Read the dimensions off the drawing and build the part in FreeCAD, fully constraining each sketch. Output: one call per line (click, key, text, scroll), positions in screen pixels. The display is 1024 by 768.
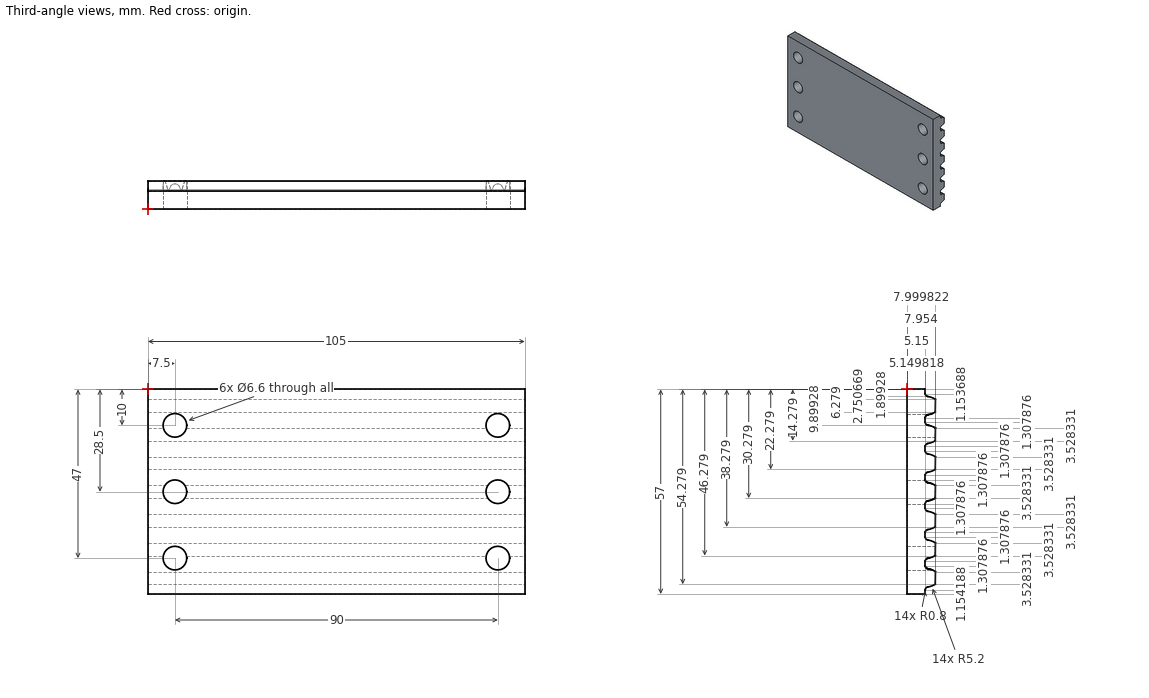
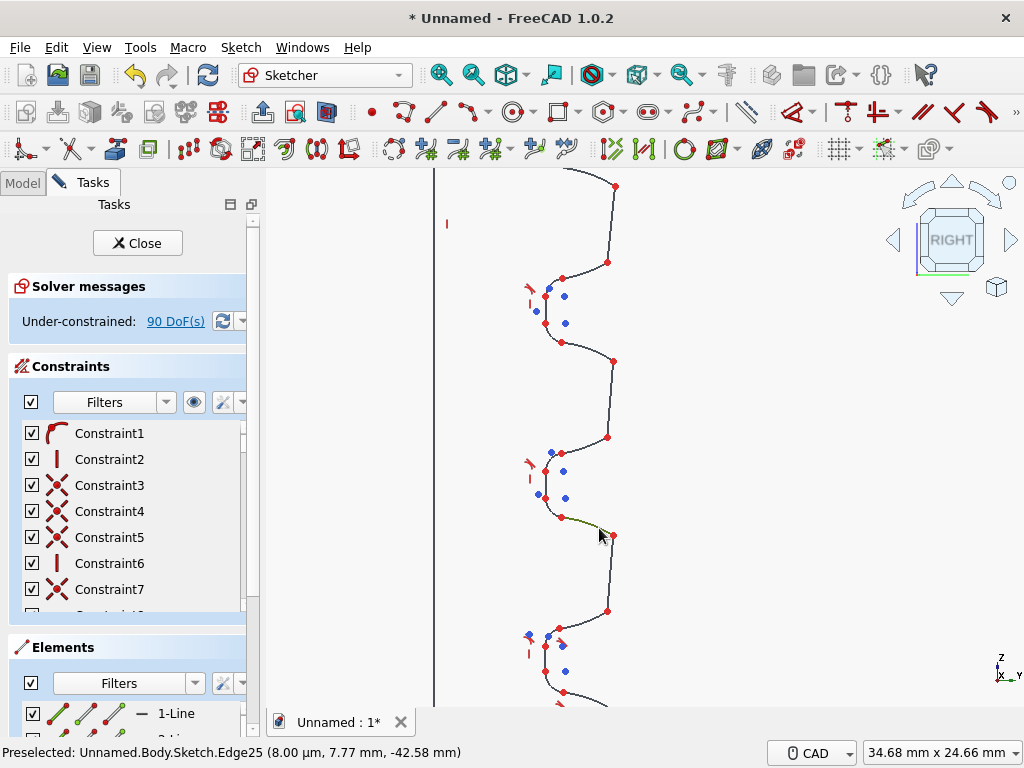
click(550, 510)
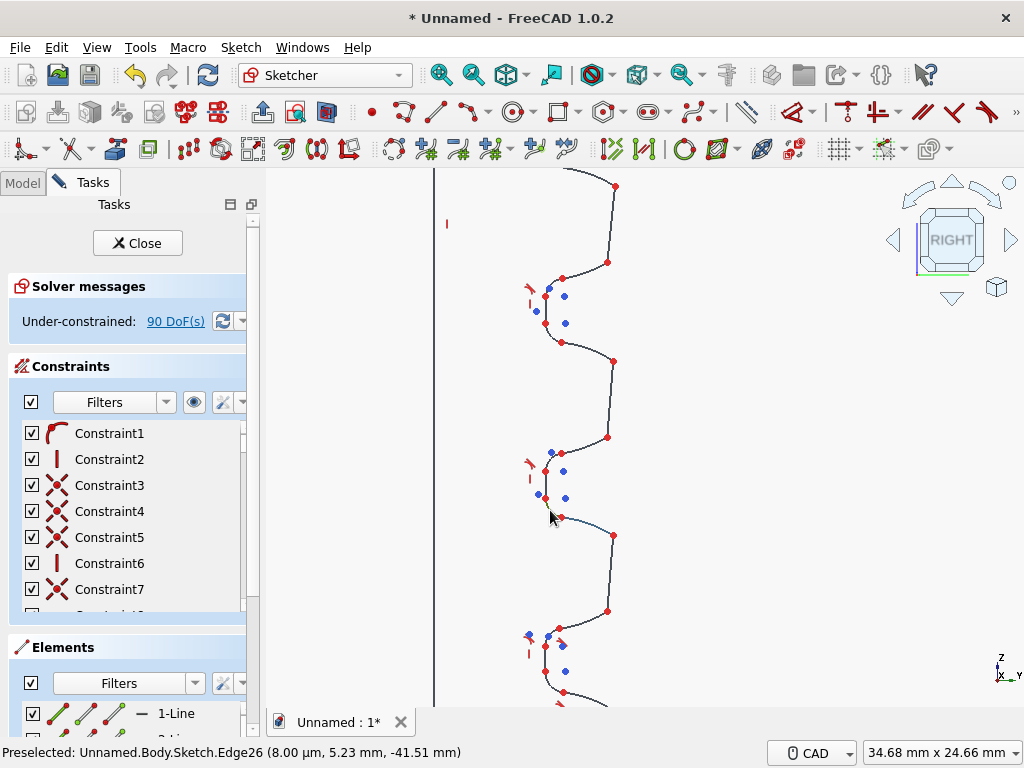
click(988, 112)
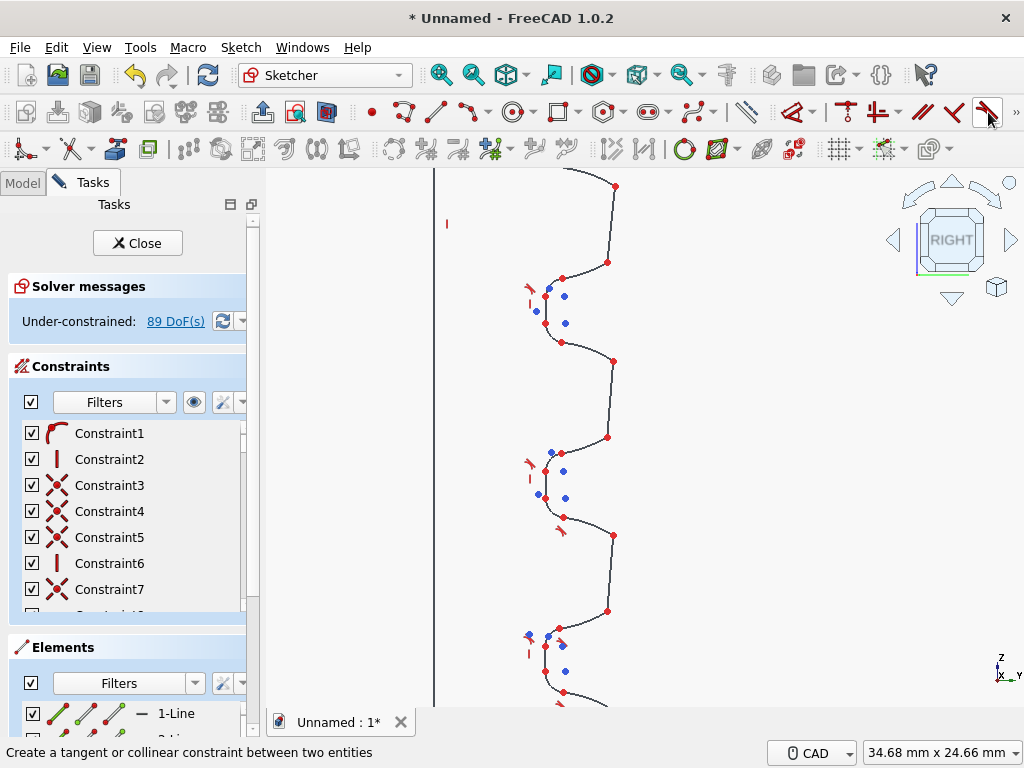
click(550, 459)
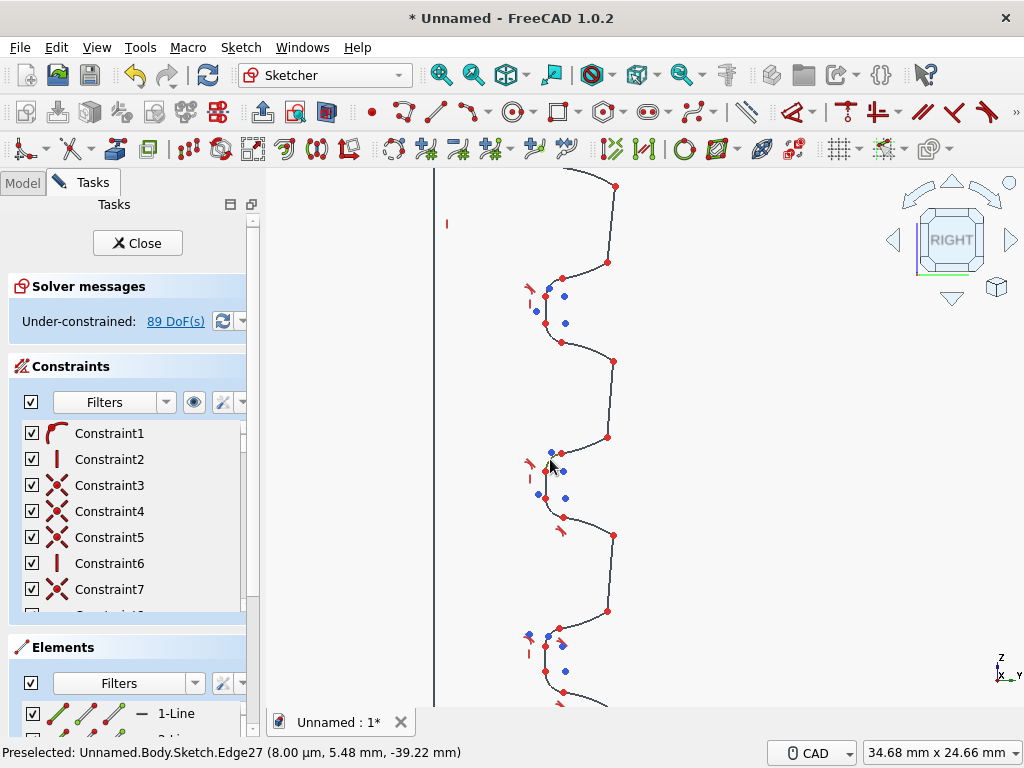
click(576, 450)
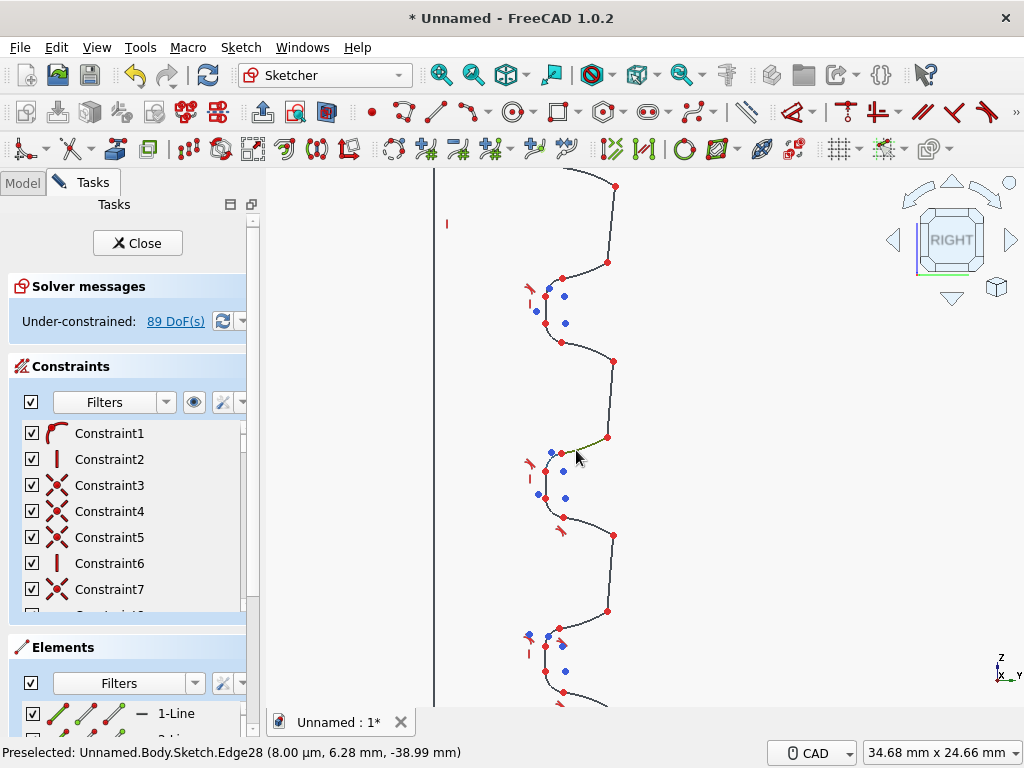
click(988, 112)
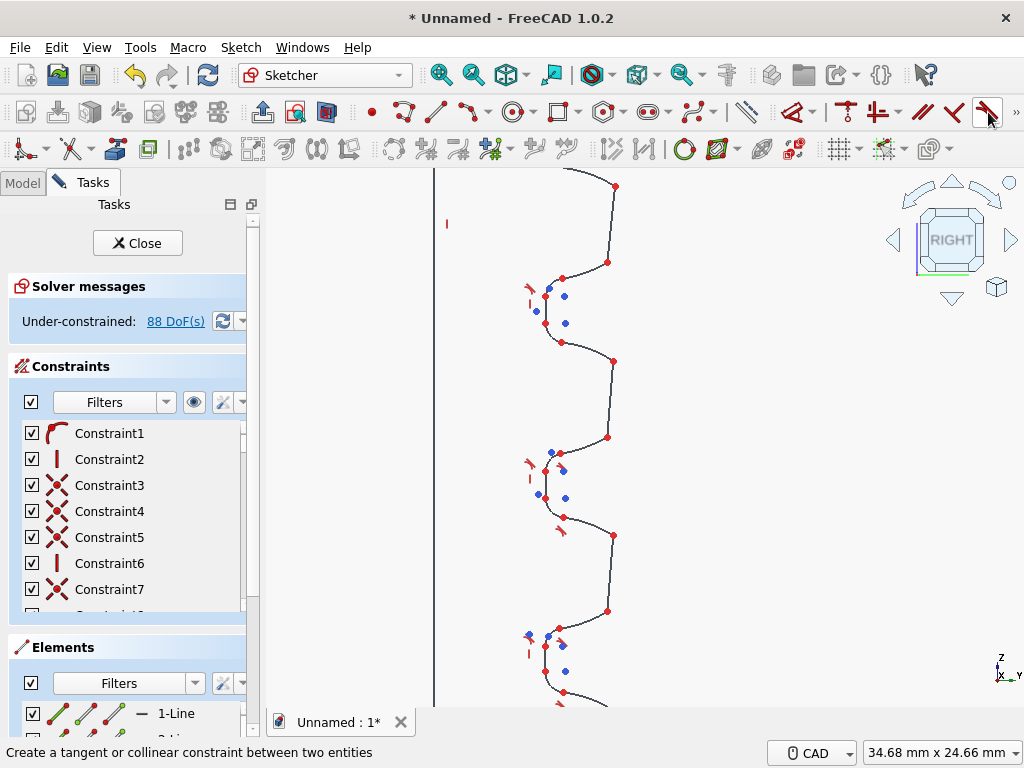
click(599, 353)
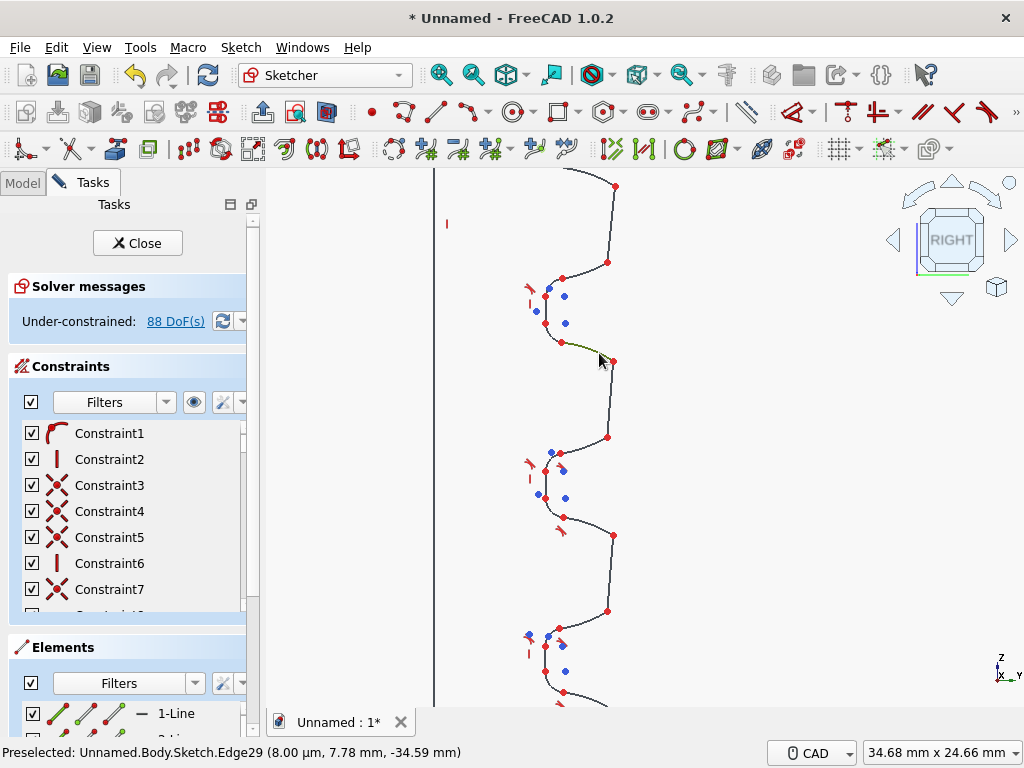
click(550, 336)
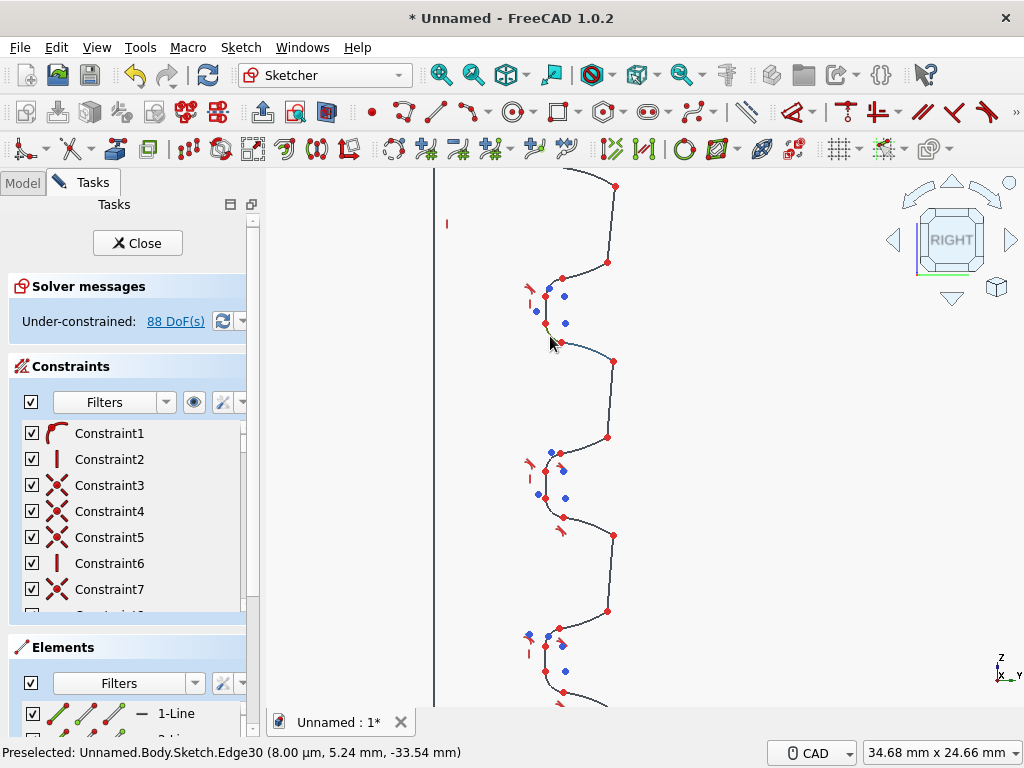
click(988, 112)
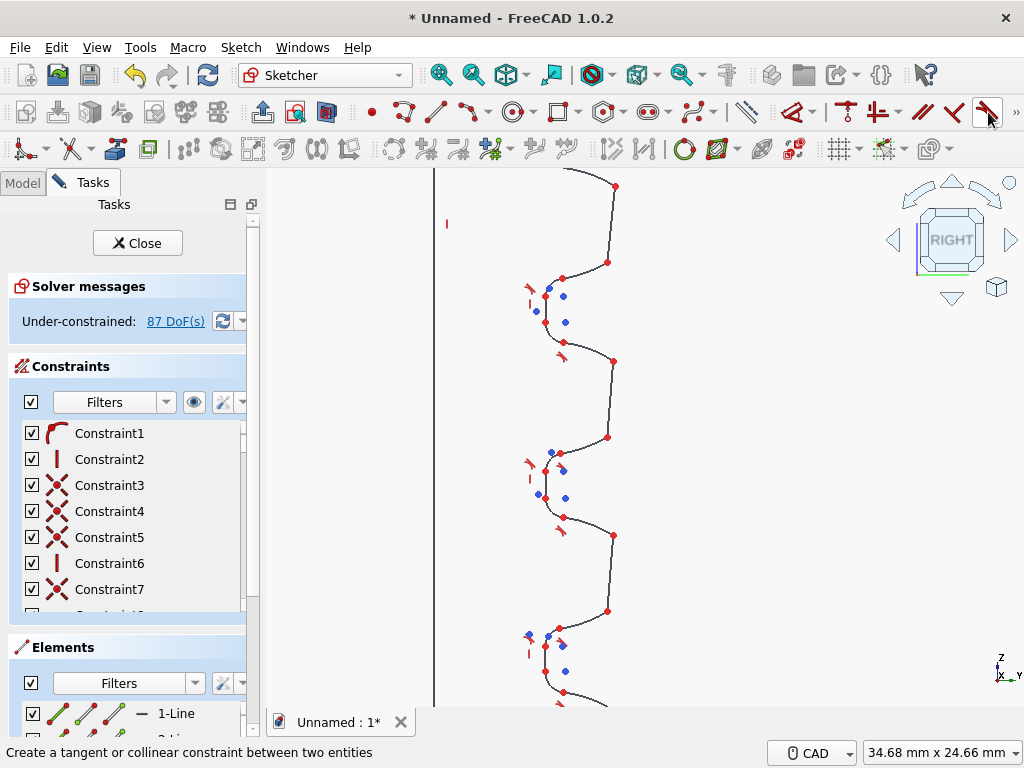
click(555, 281)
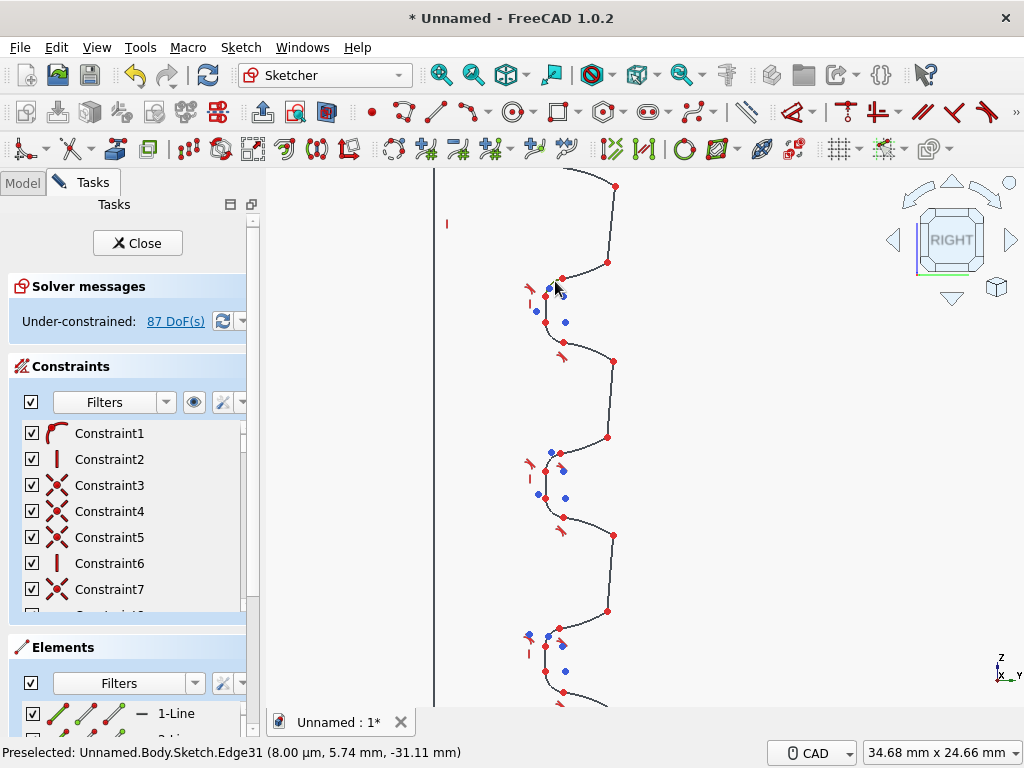
click(576, 276)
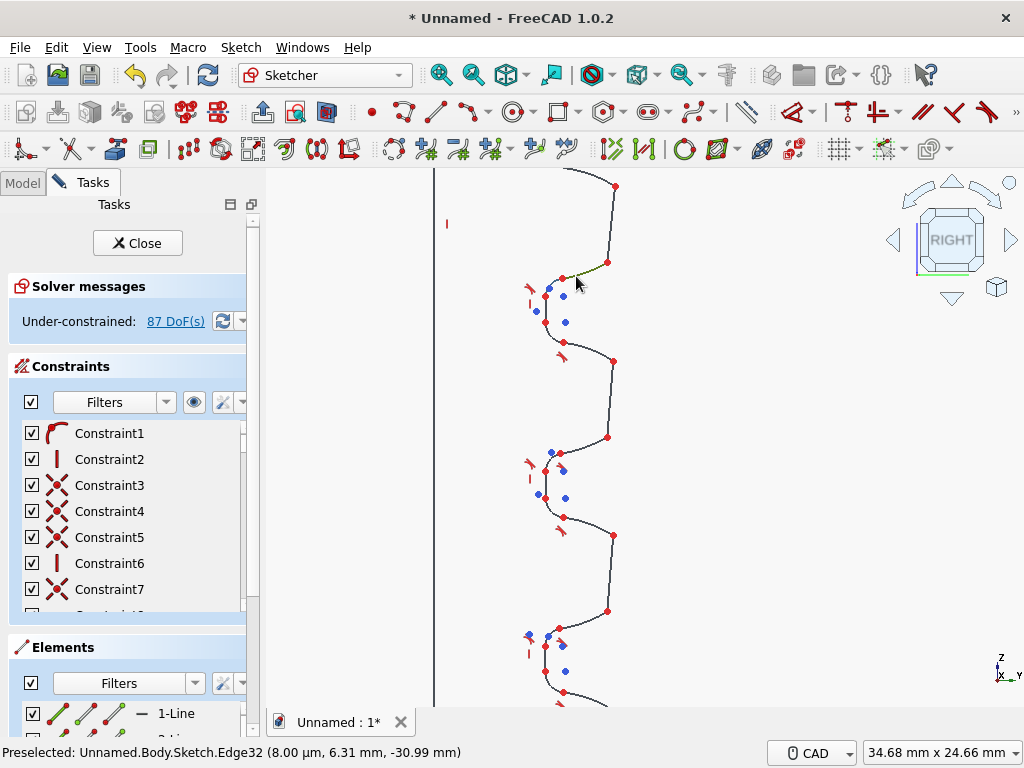
click(988, 112)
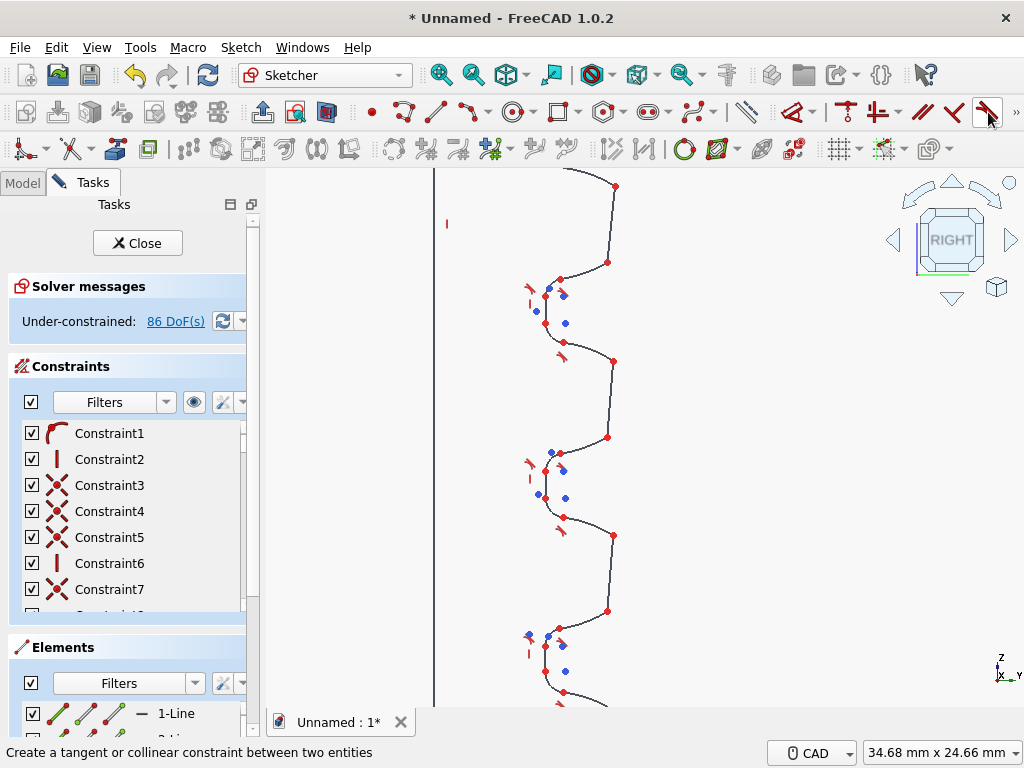
scroll(600, 530, down, 6)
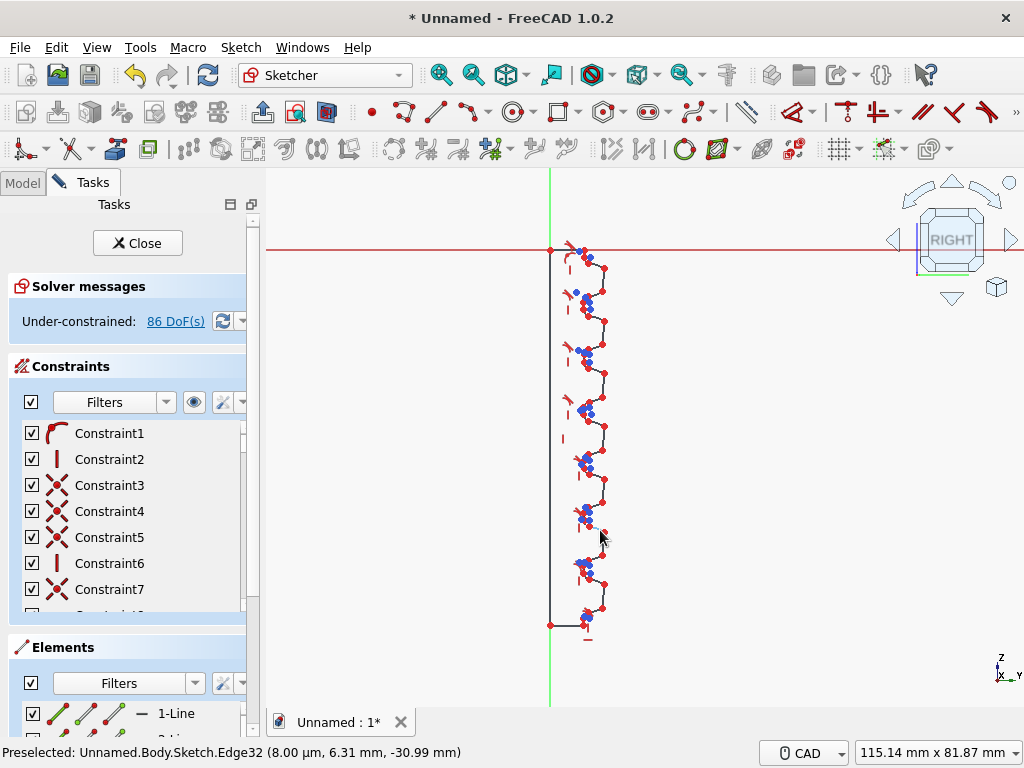
scroll(600, 425, up, 5)